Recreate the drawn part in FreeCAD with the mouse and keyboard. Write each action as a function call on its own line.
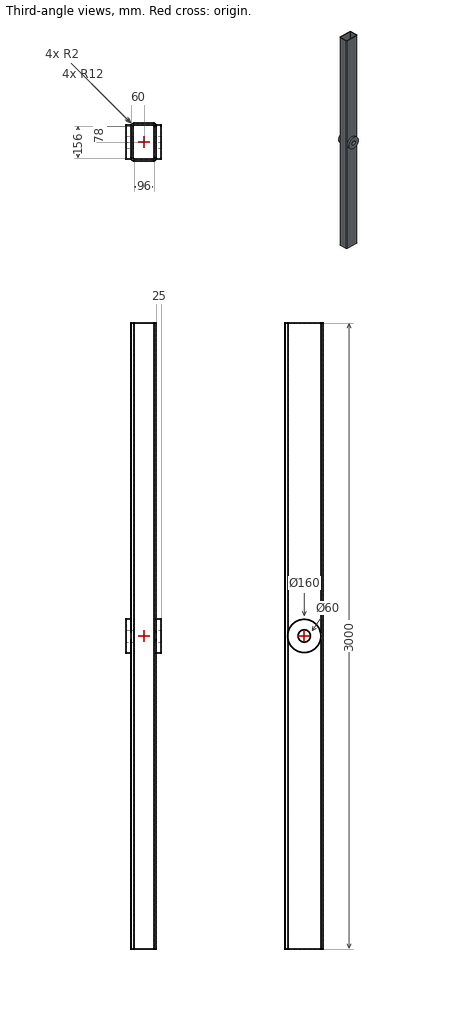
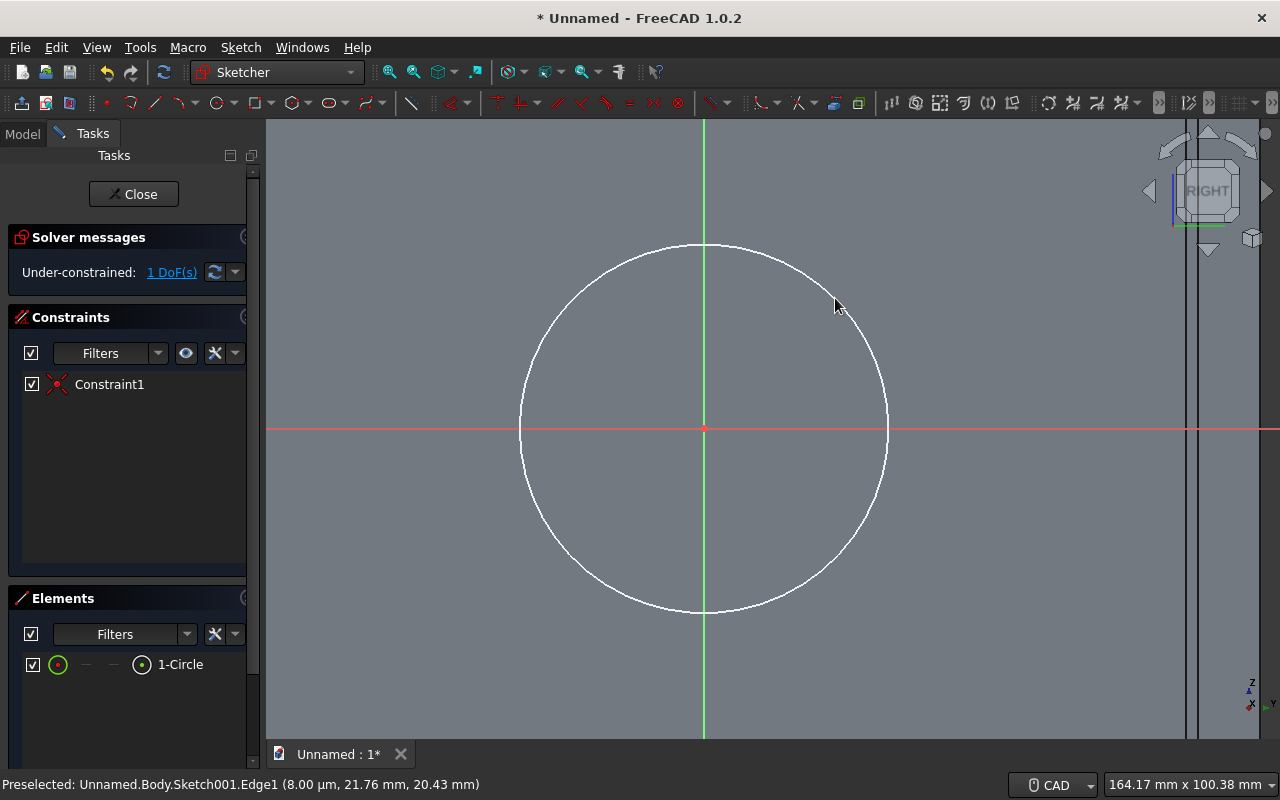
click(450, 104)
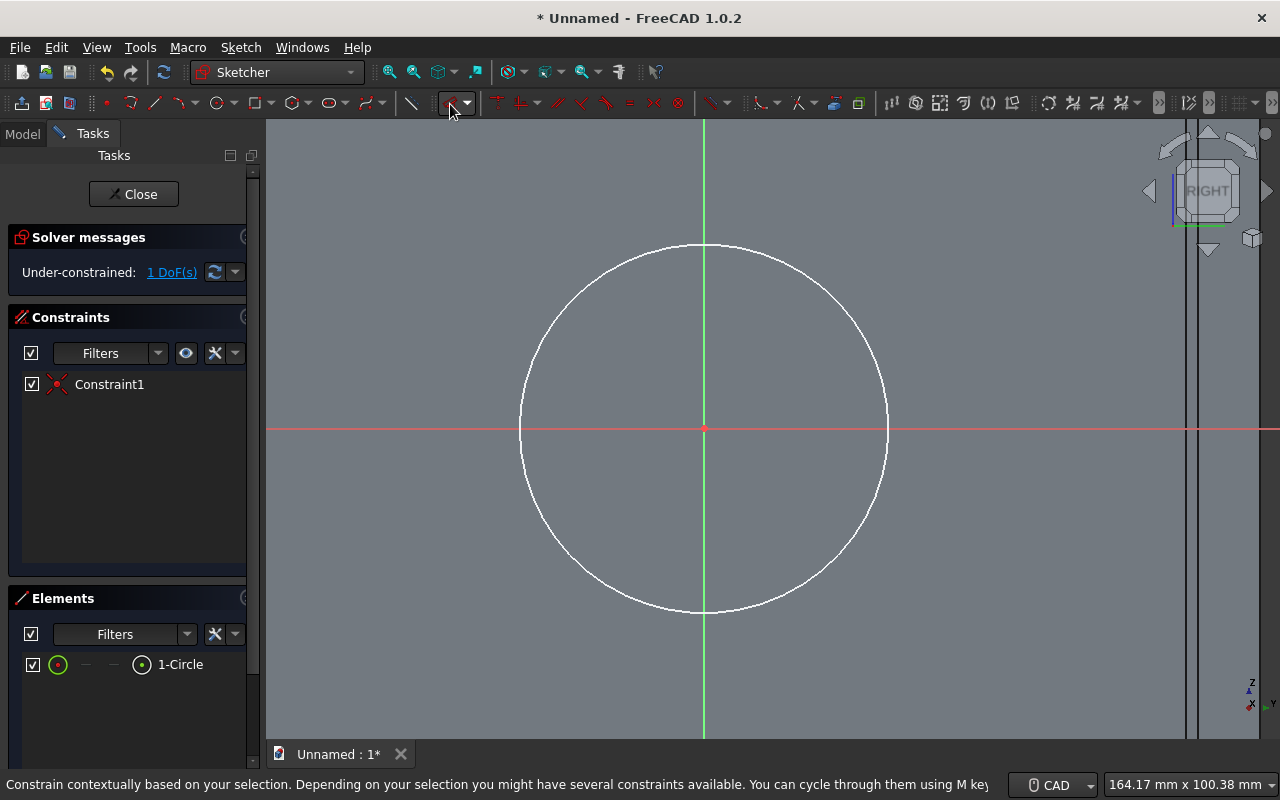
click(834, 298)
click(857, 275)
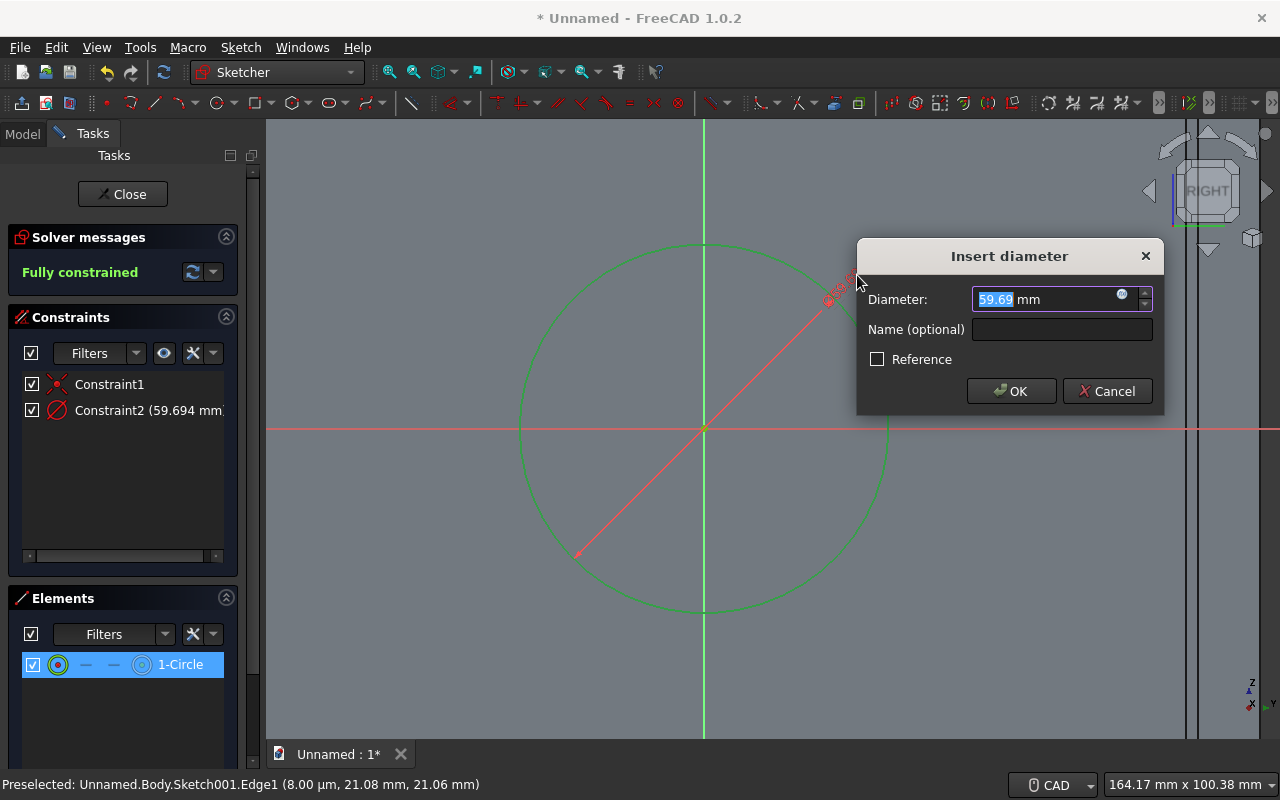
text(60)
key(Return)
key(Escape)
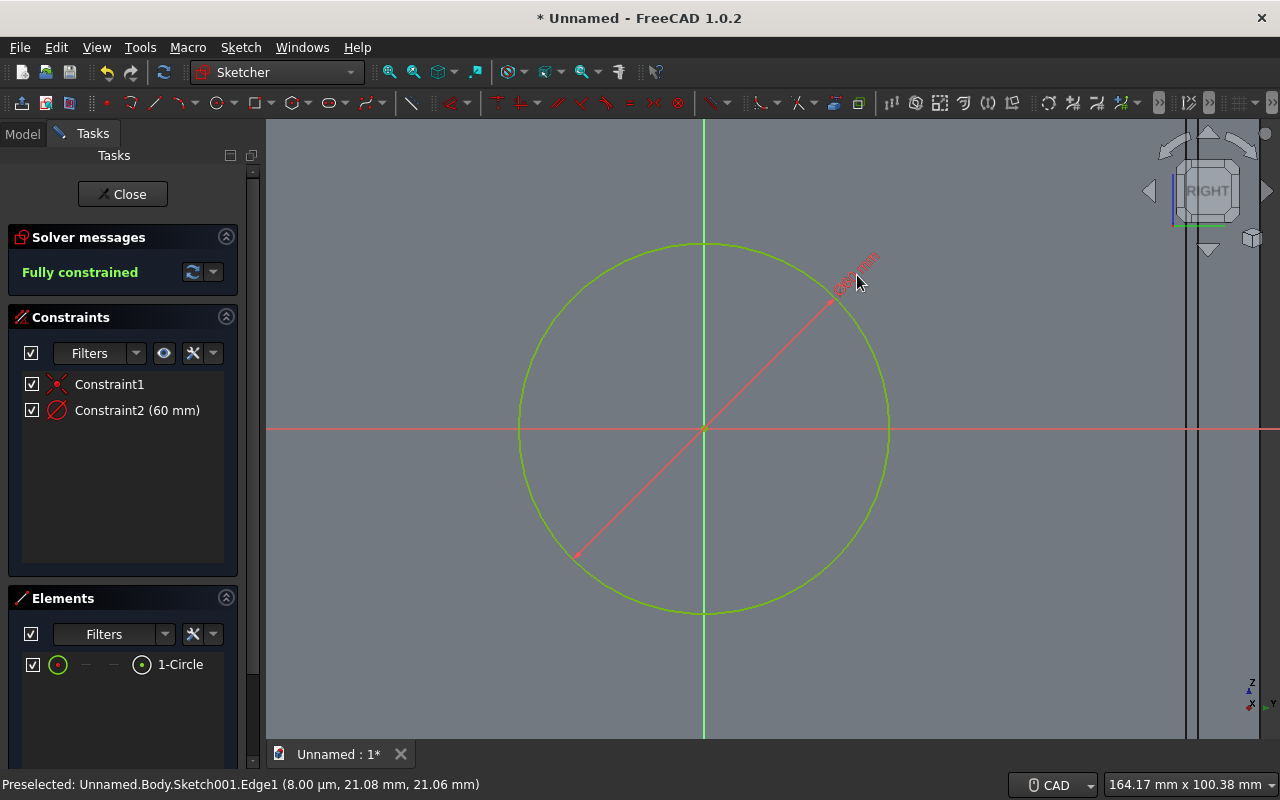
click(123, 194)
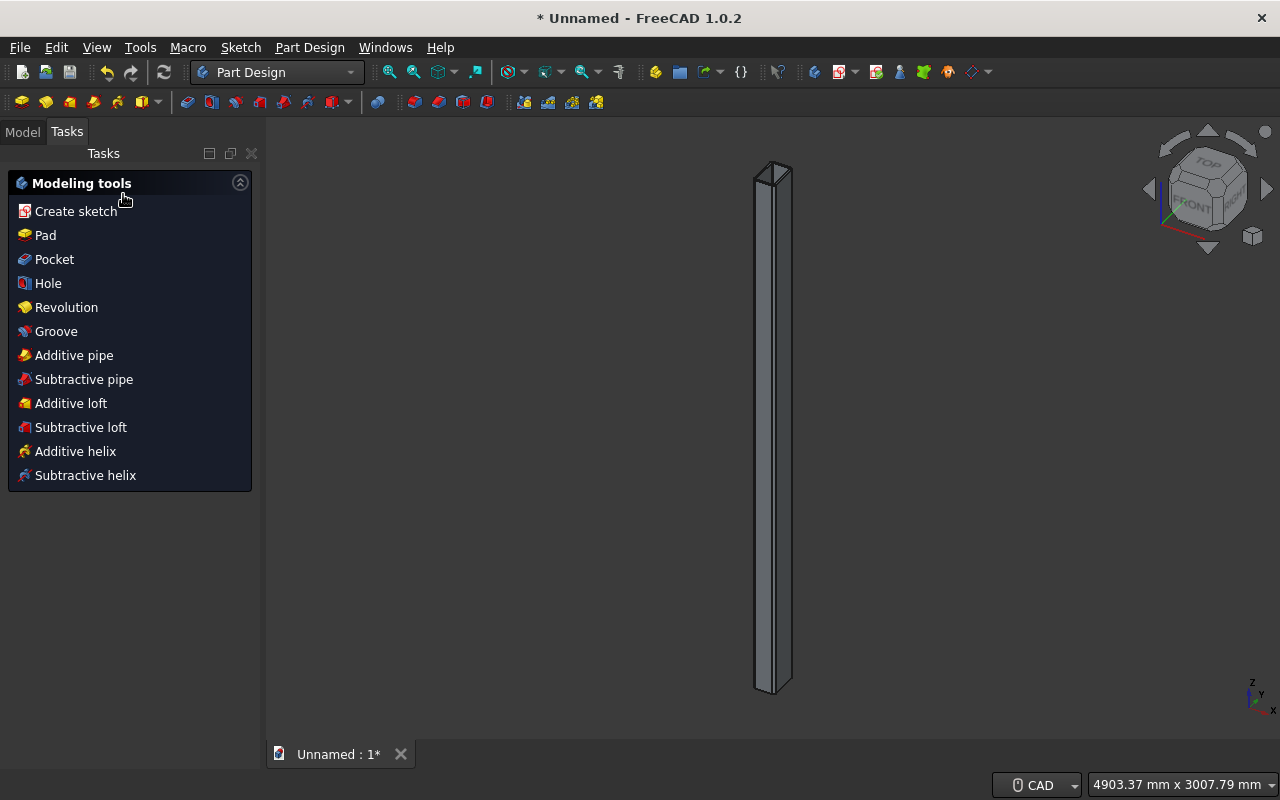
click(188, 102)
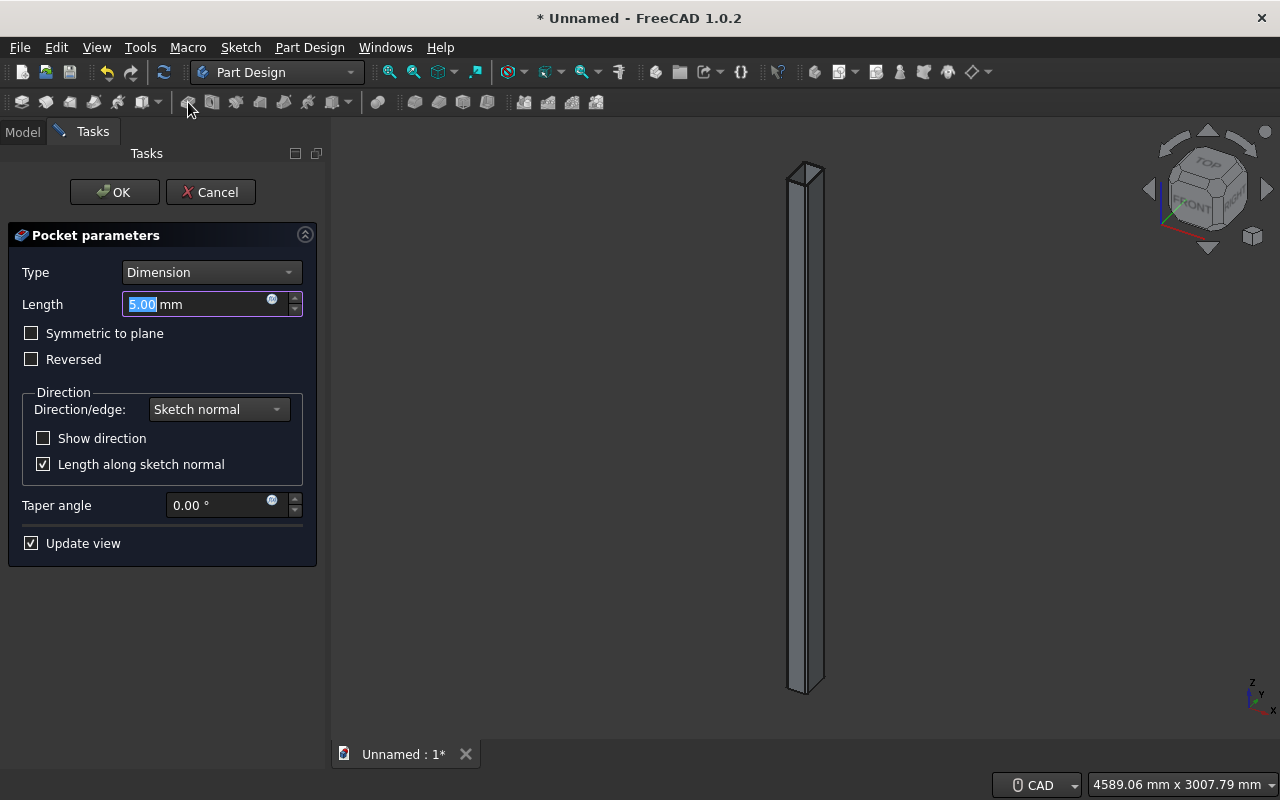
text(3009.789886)
key(Tab)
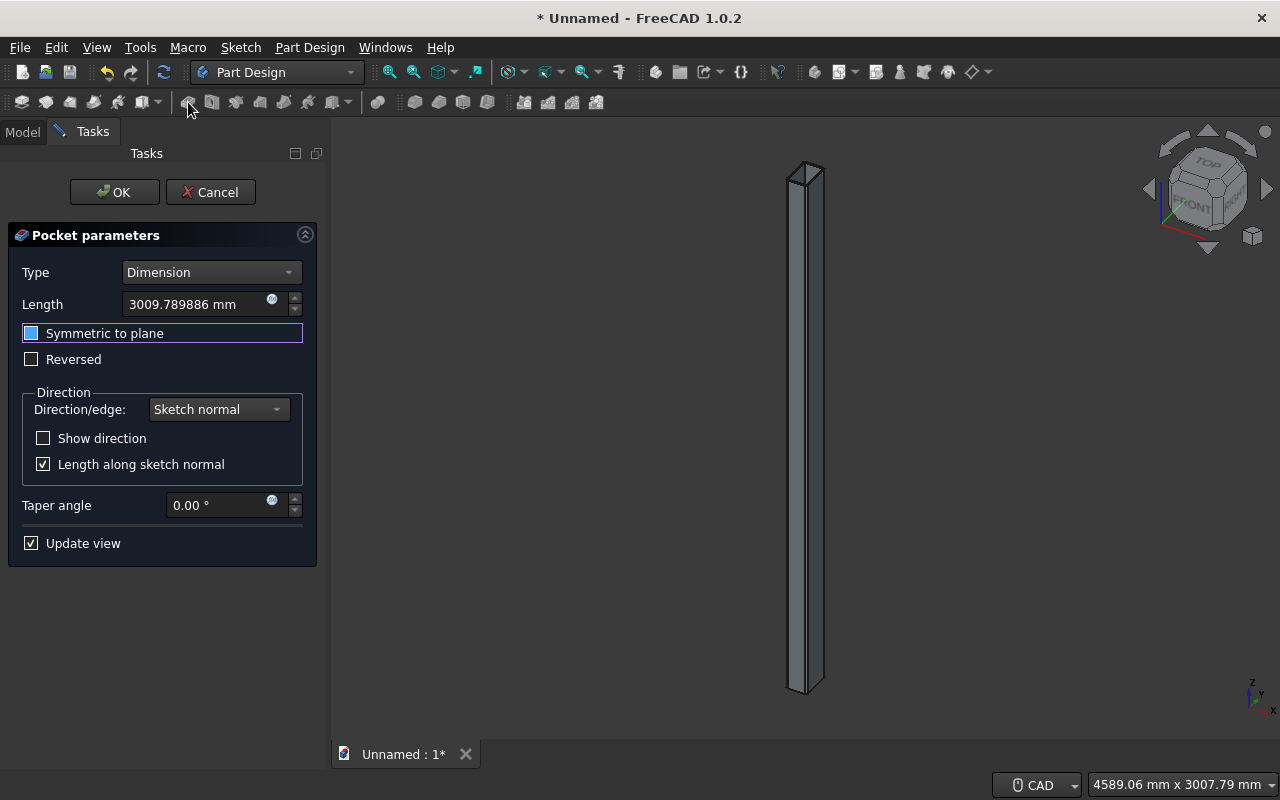
click(30, 333)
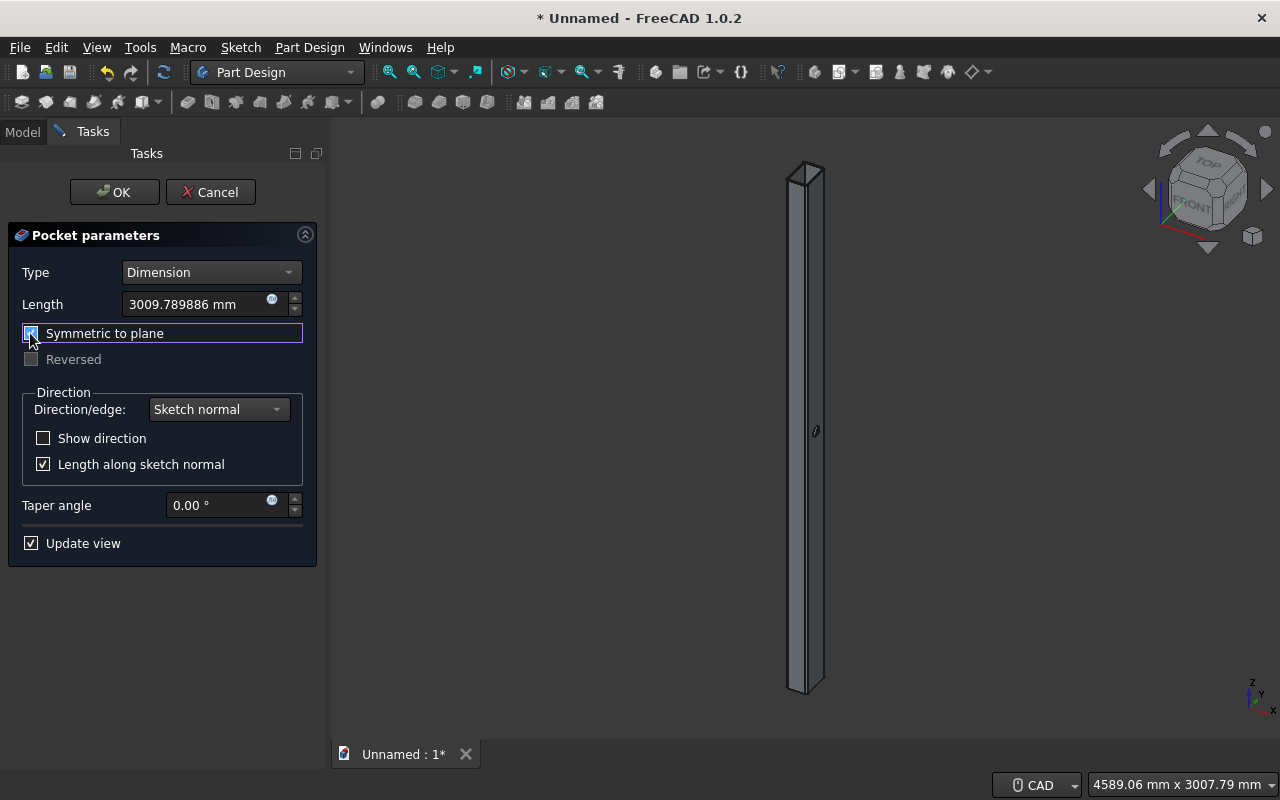
click(115, 192)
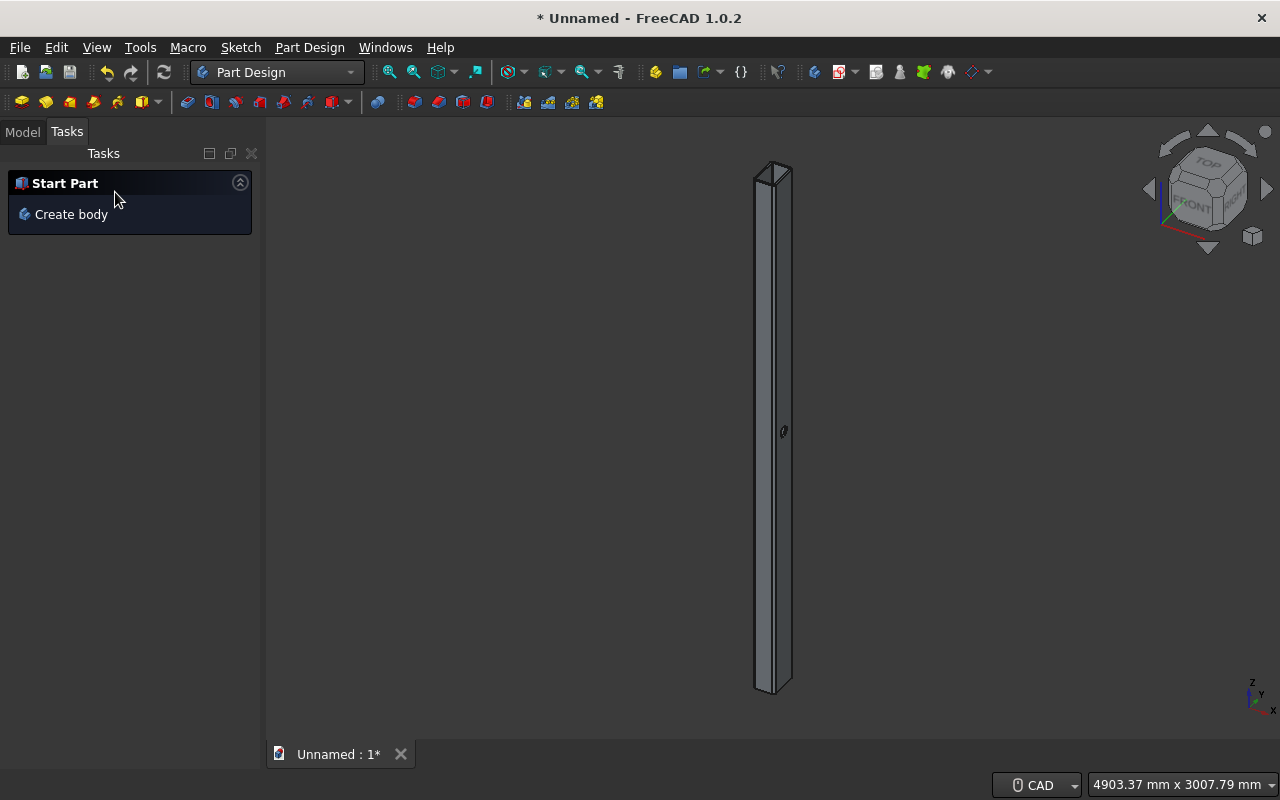
click(784, 213)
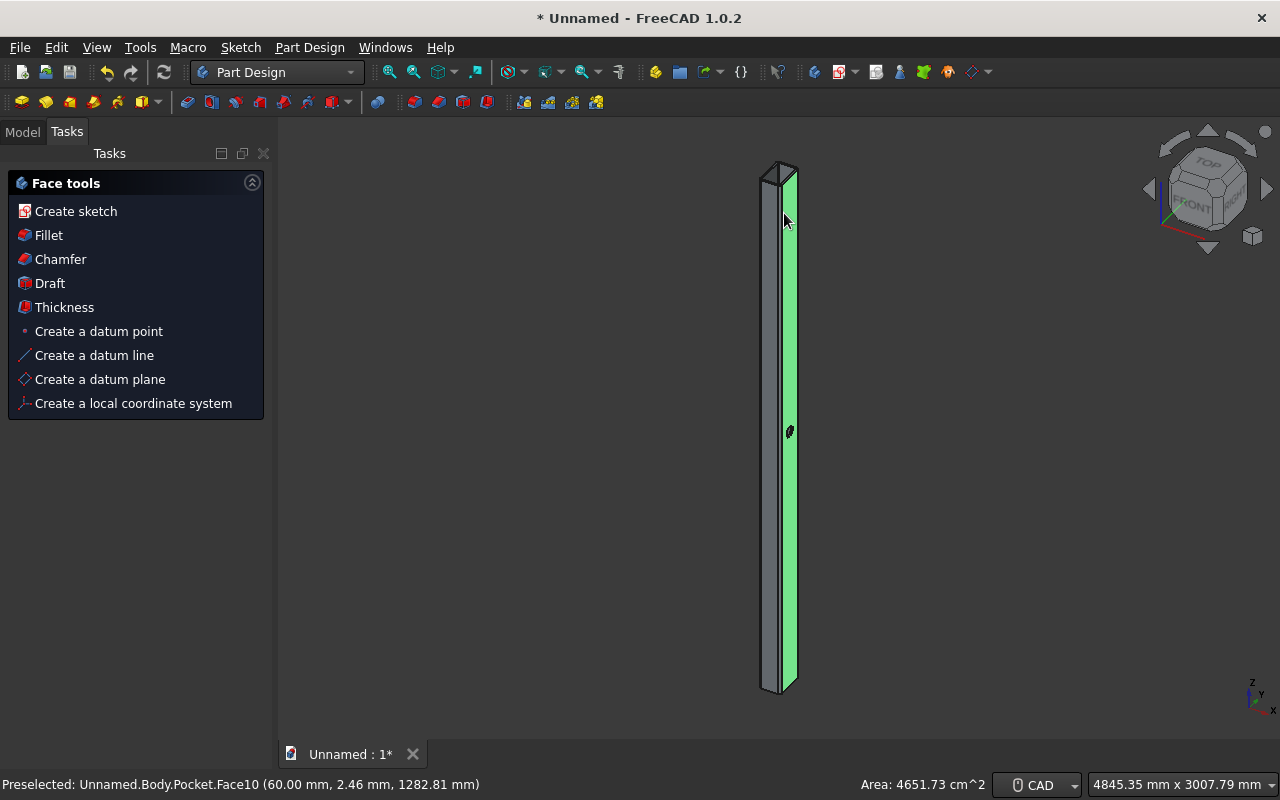
click(840, 72)